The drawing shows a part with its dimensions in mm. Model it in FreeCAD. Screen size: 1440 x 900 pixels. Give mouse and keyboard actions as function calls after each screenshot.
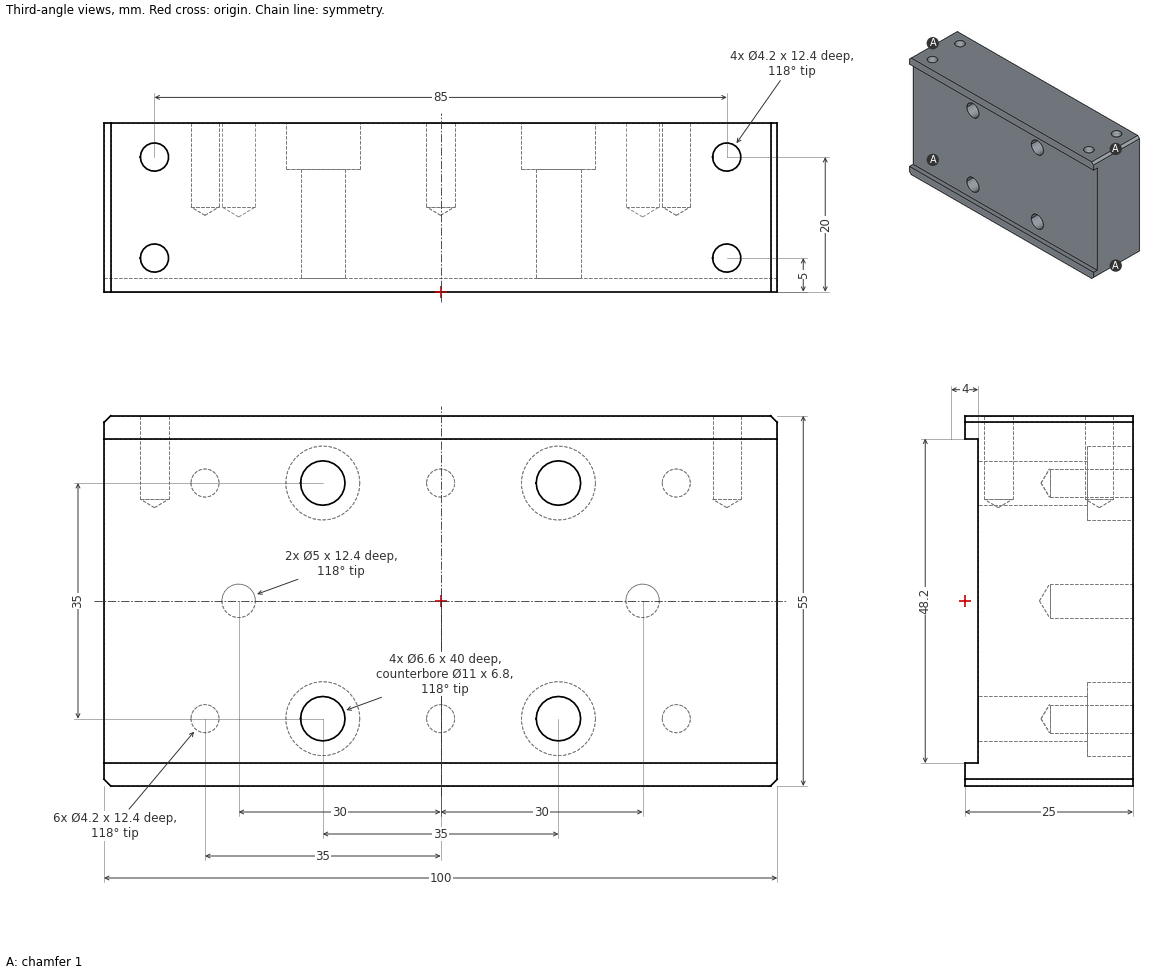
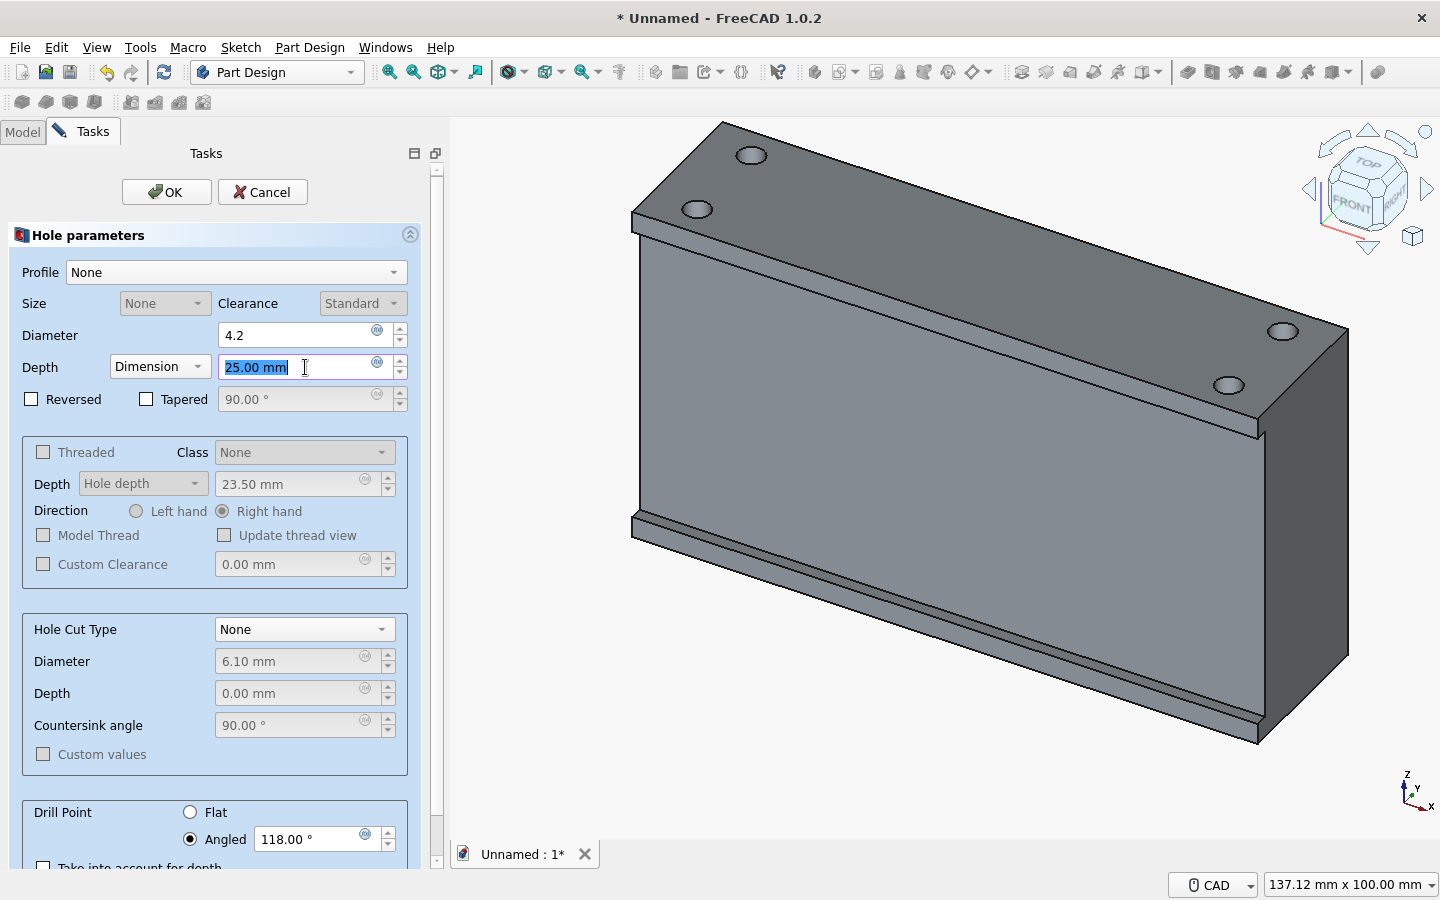
text(12.4)
key(Tab)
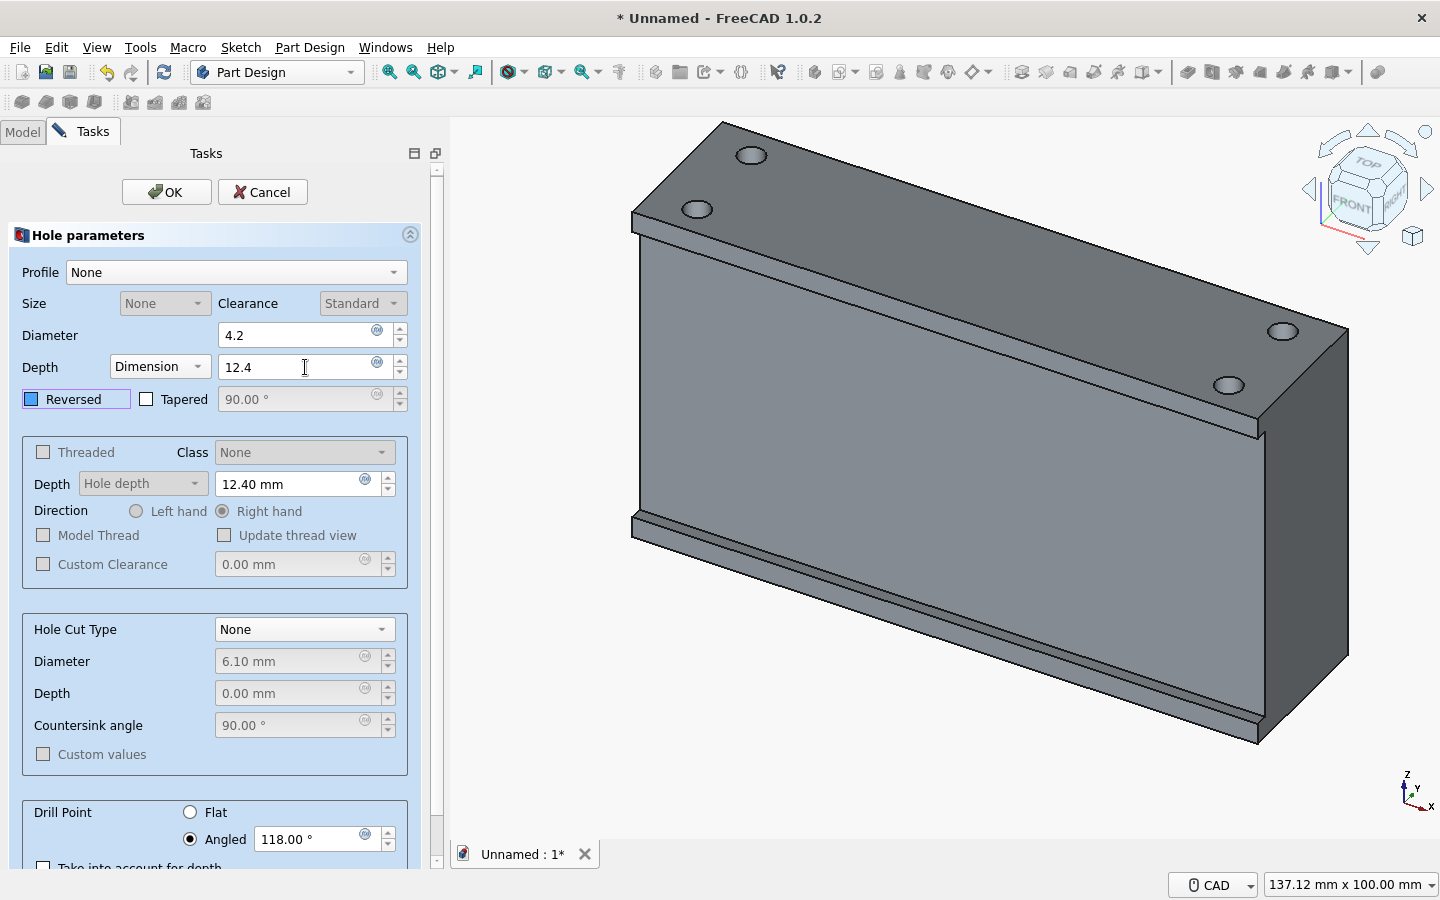
click(167, 192)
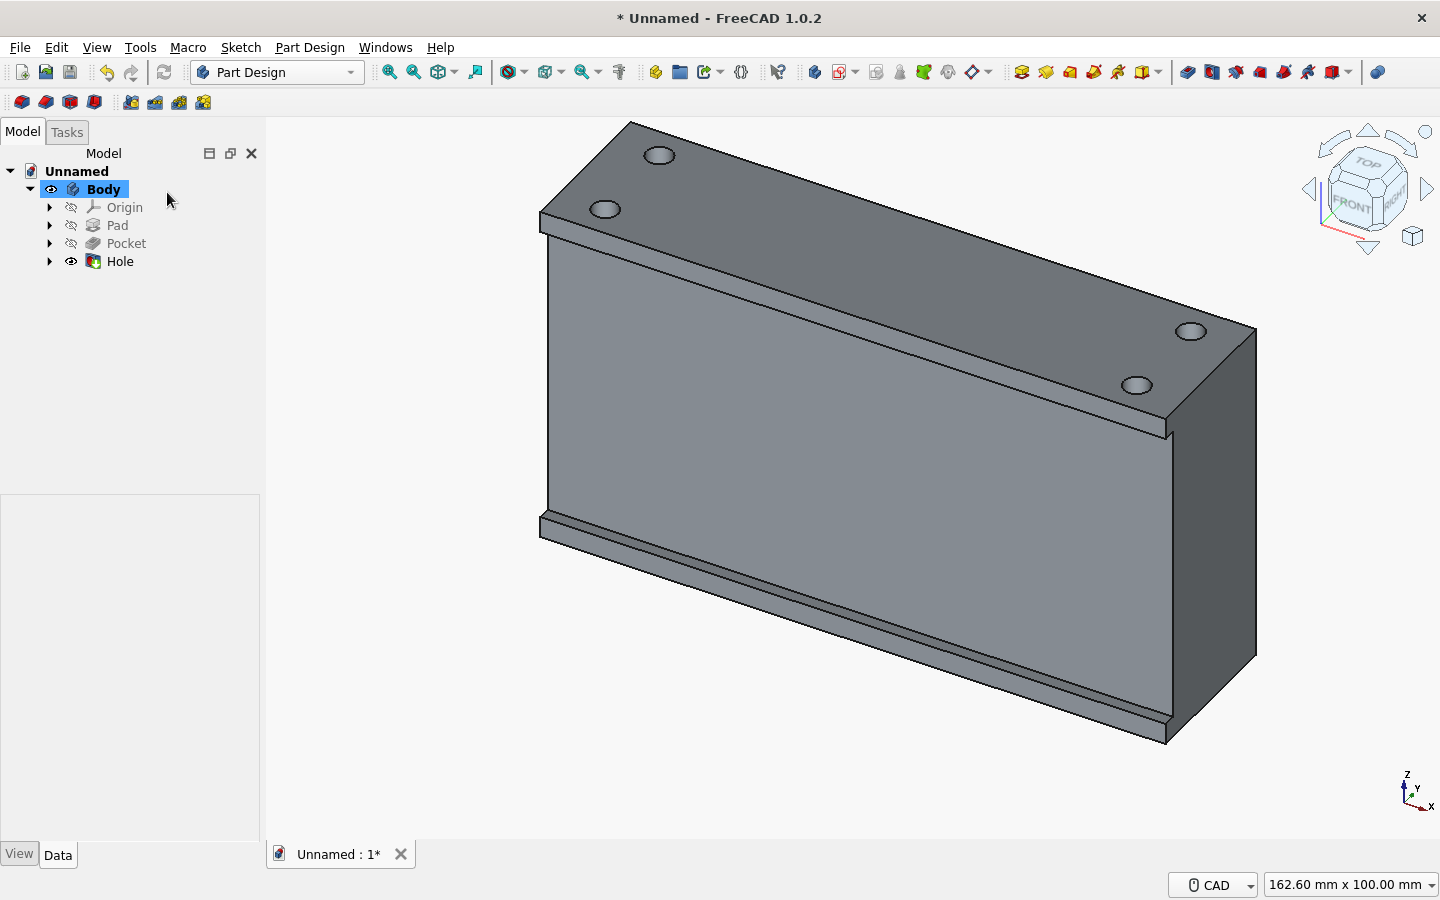
click(1211, 373)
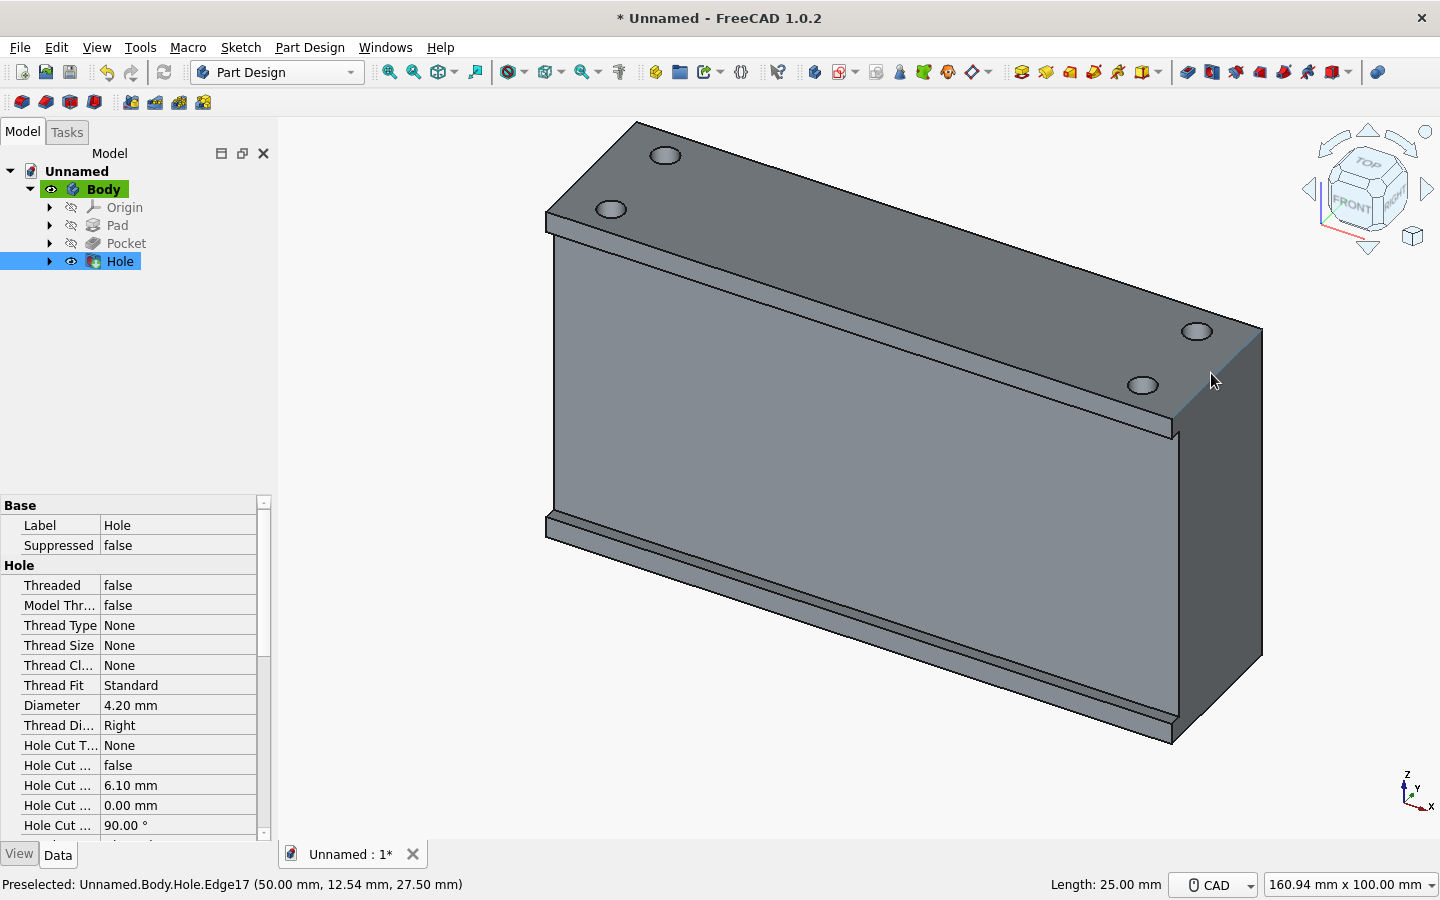
key(0)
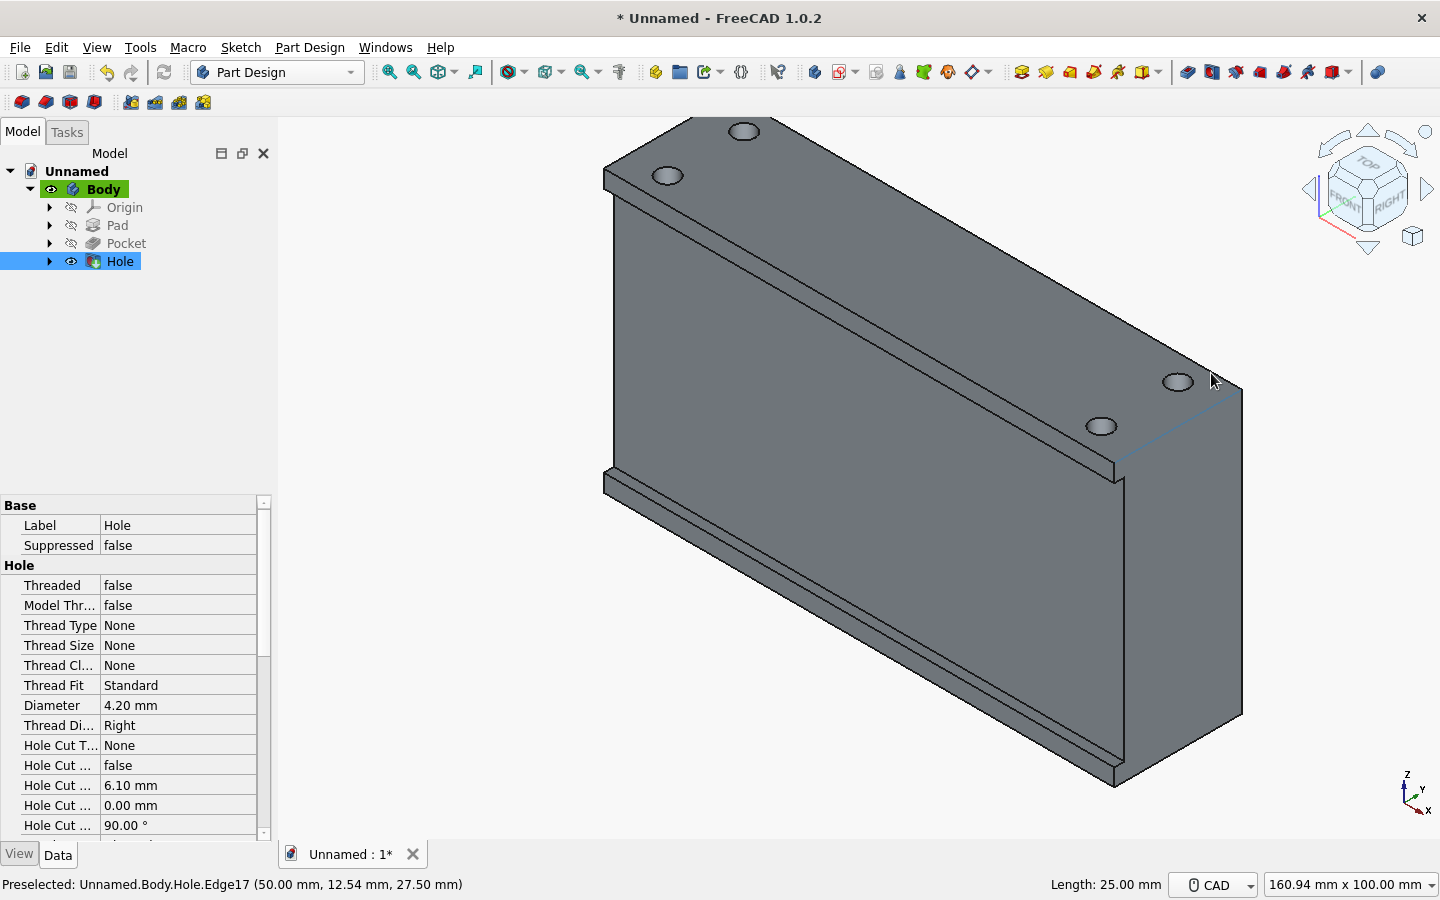
click(390, 72)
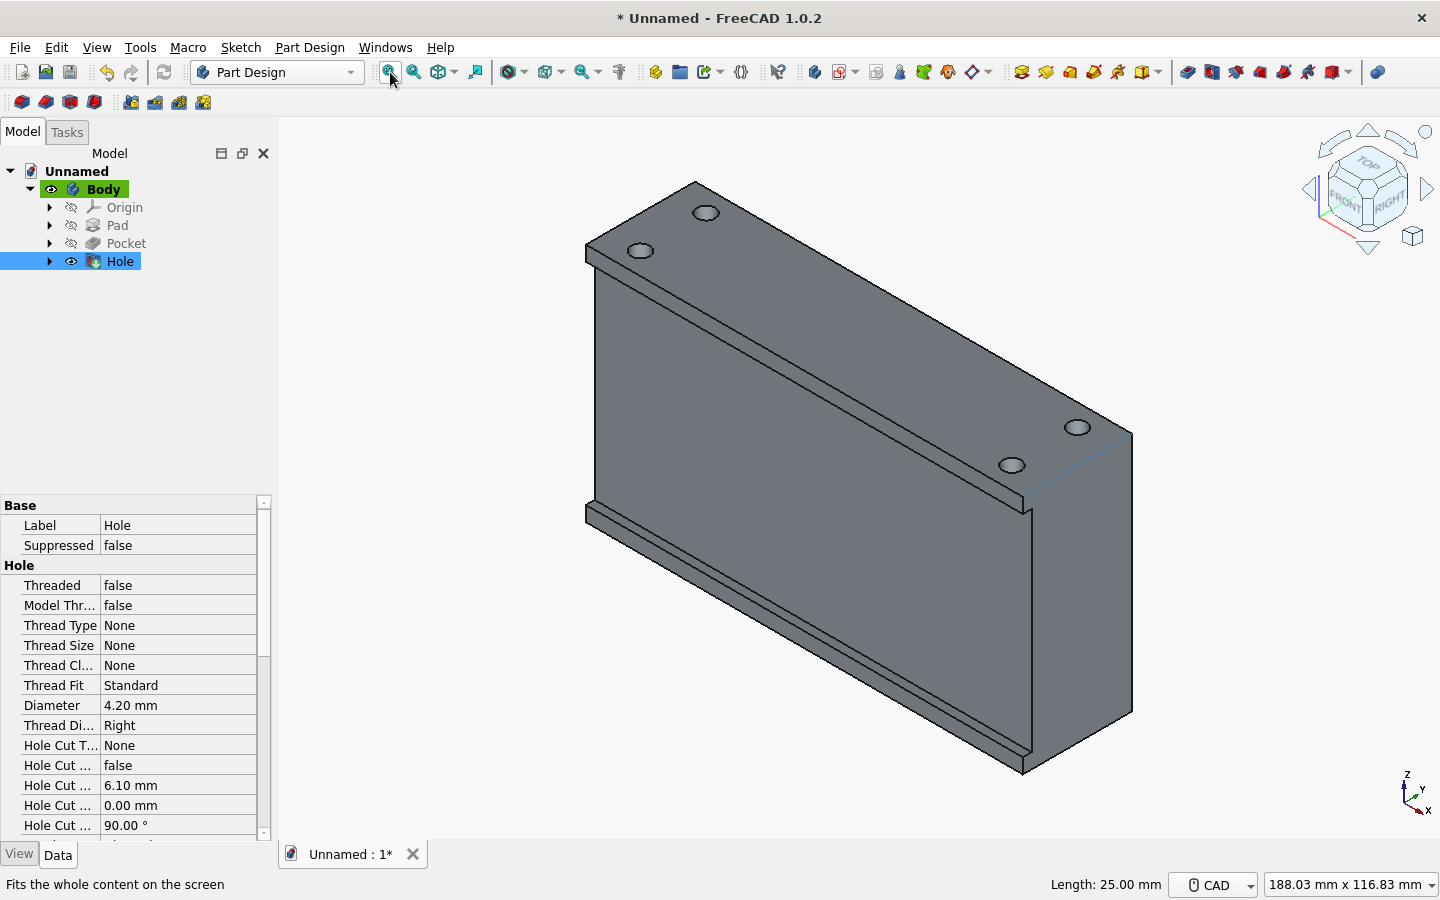
key(2)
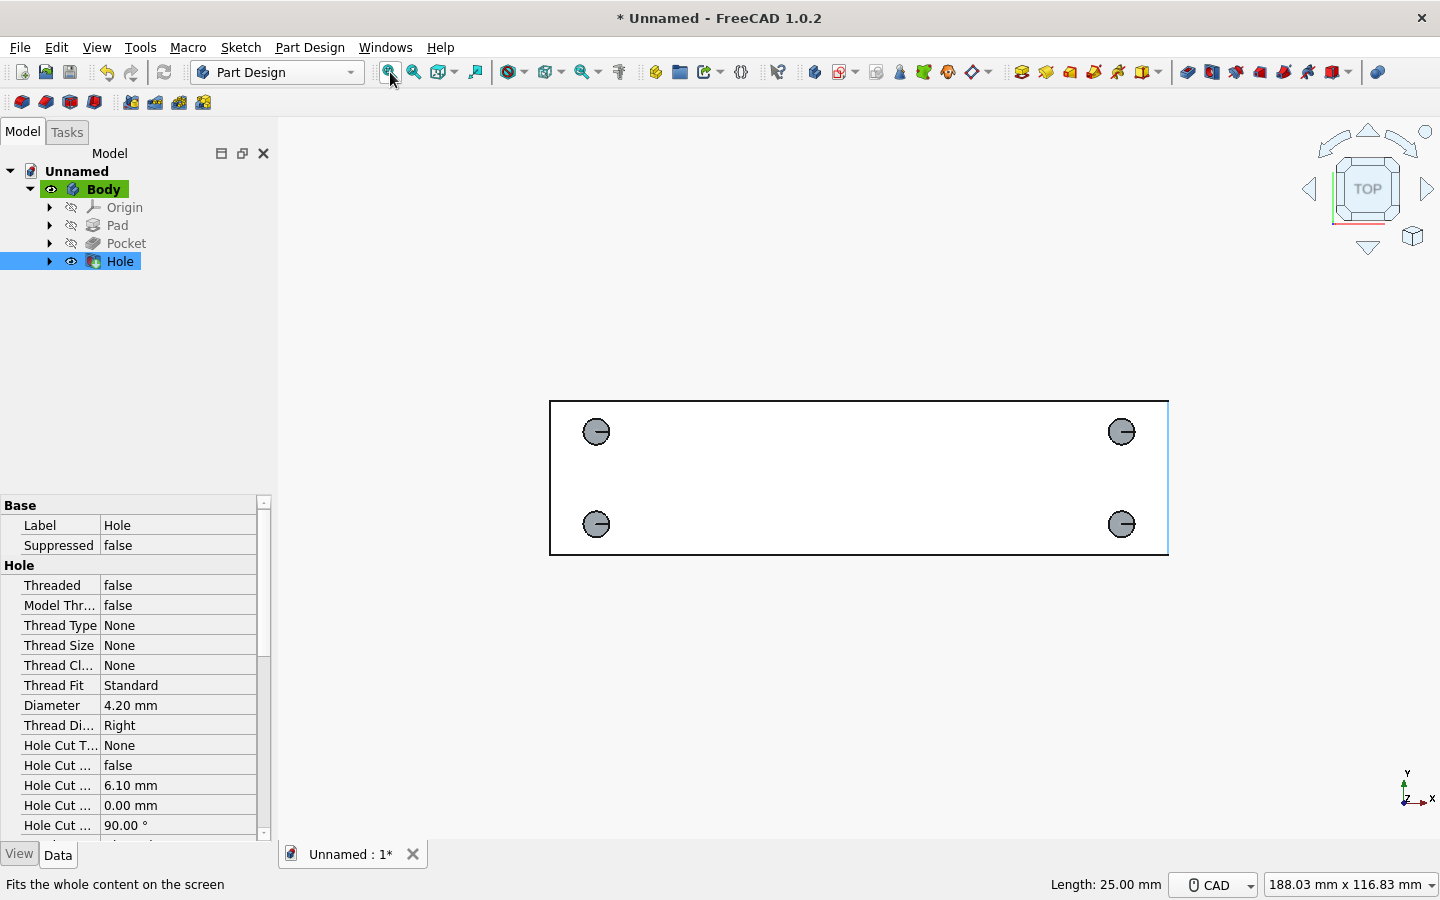
click(550, 477, ctrl)